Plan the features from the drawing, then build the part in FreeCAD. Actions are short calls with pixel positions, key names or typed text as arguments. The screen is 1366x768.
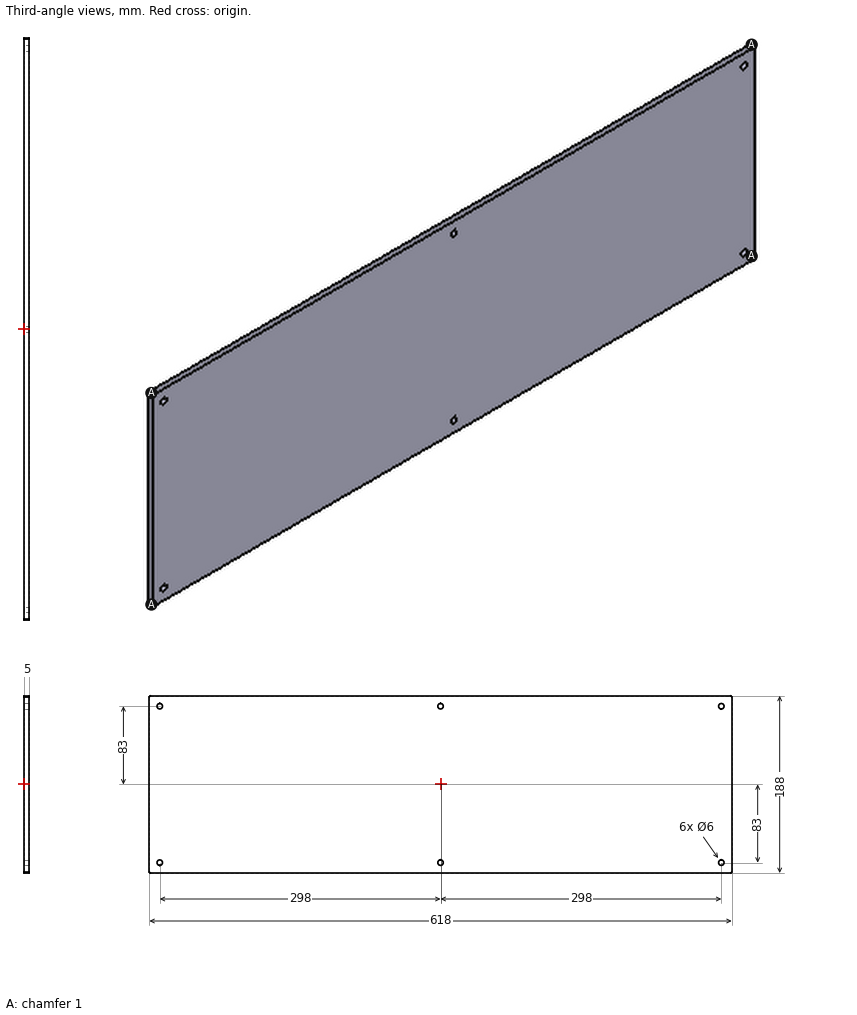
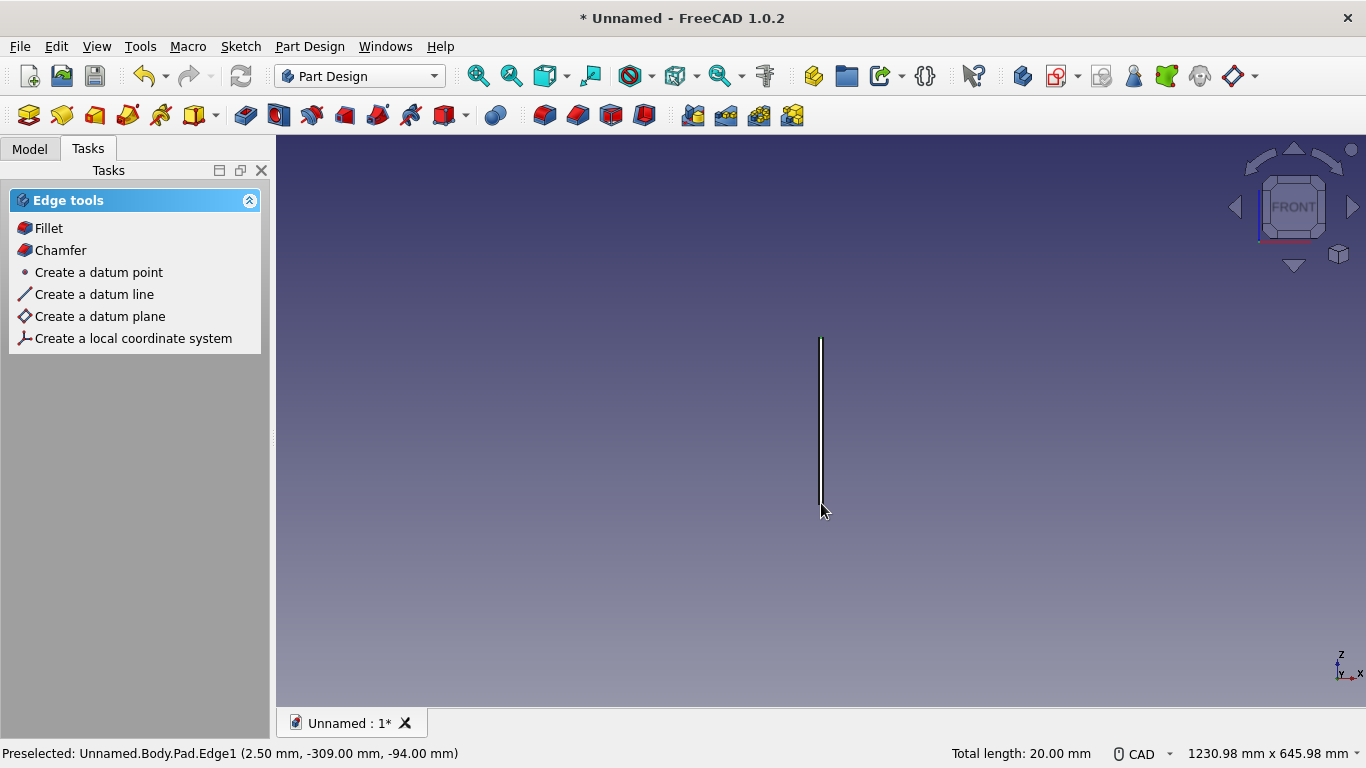
click(578, 116)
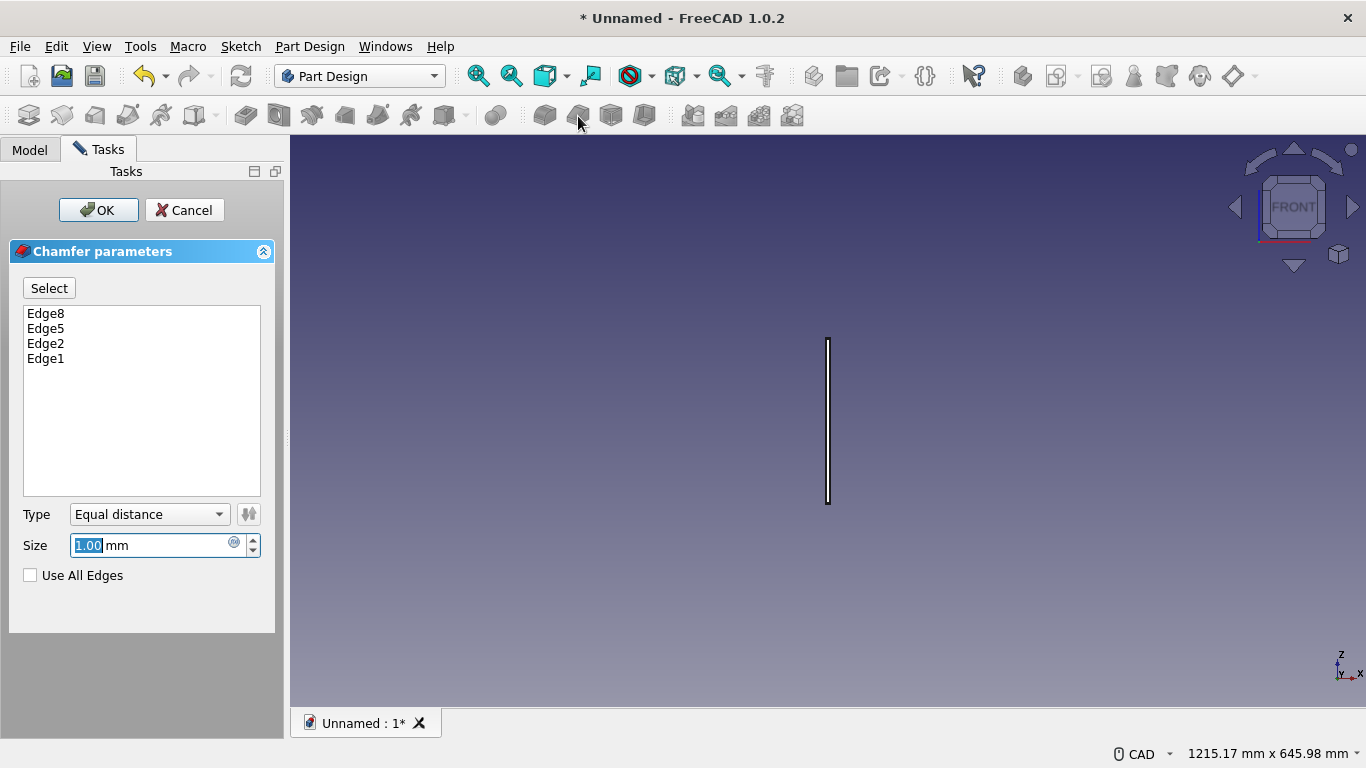
text(1)
key(Tab)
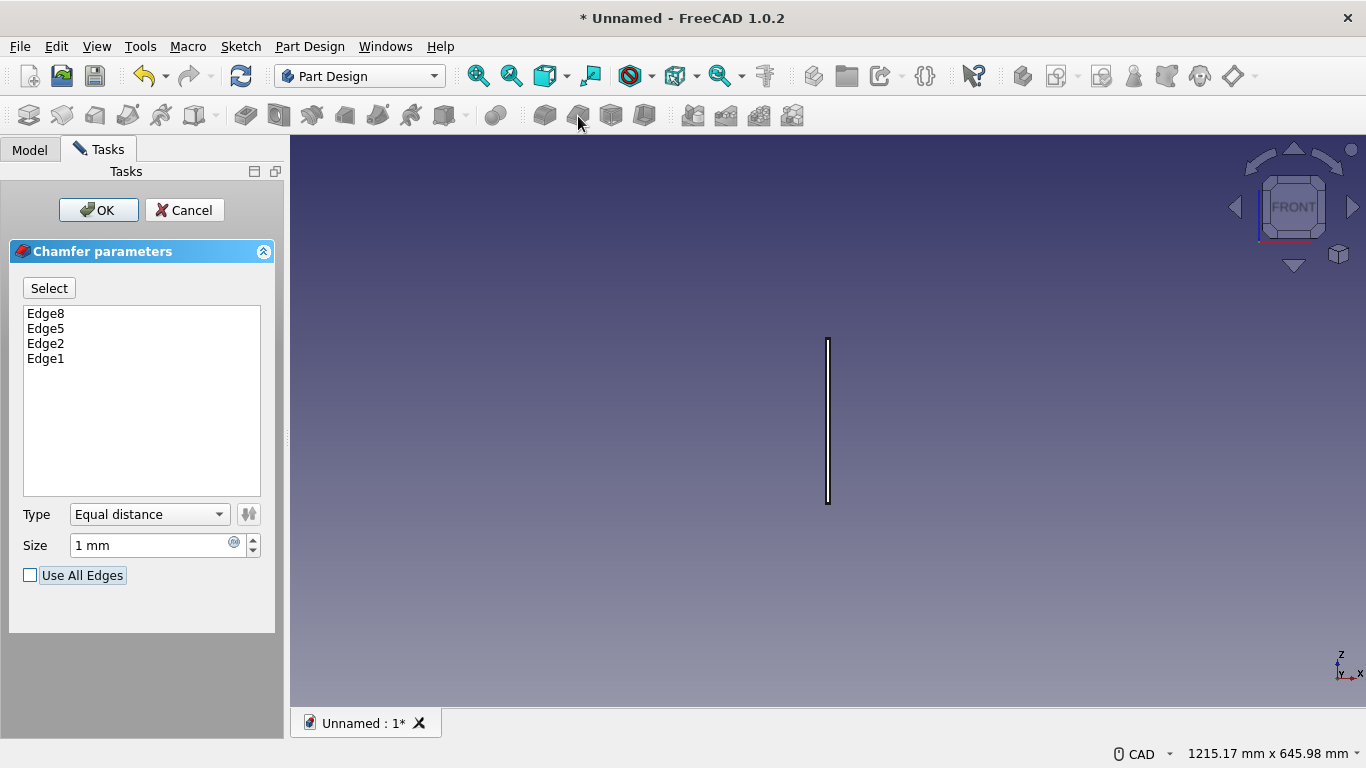
click(99, 210)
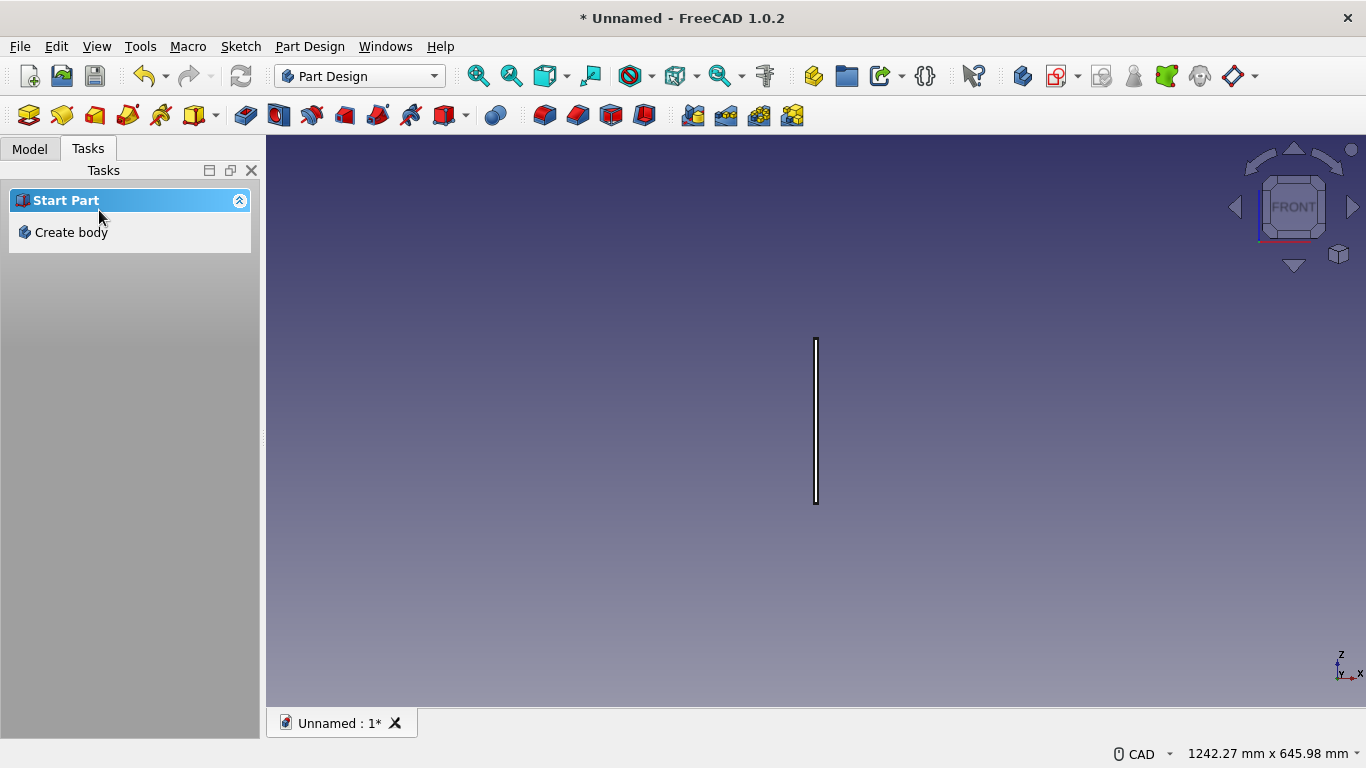
click(479, 76)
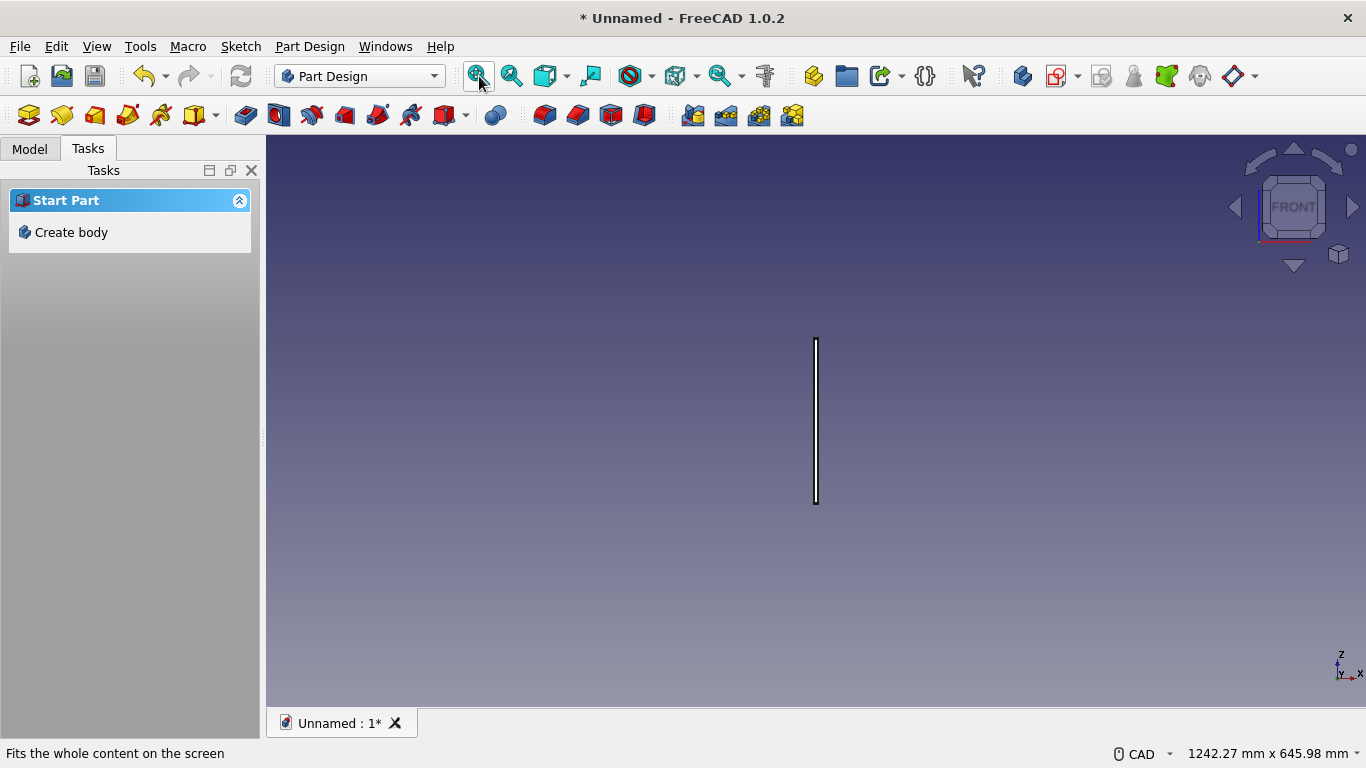
key(6)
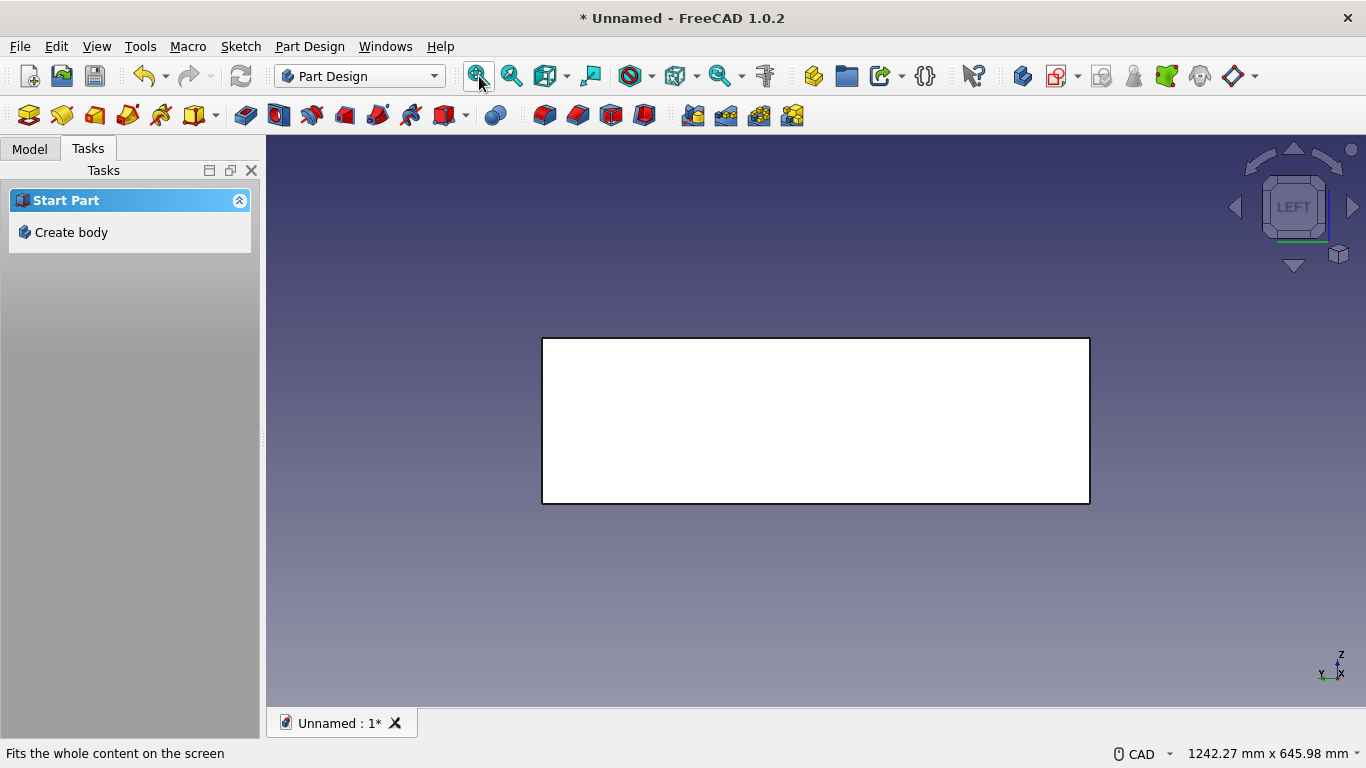
click(660, 420)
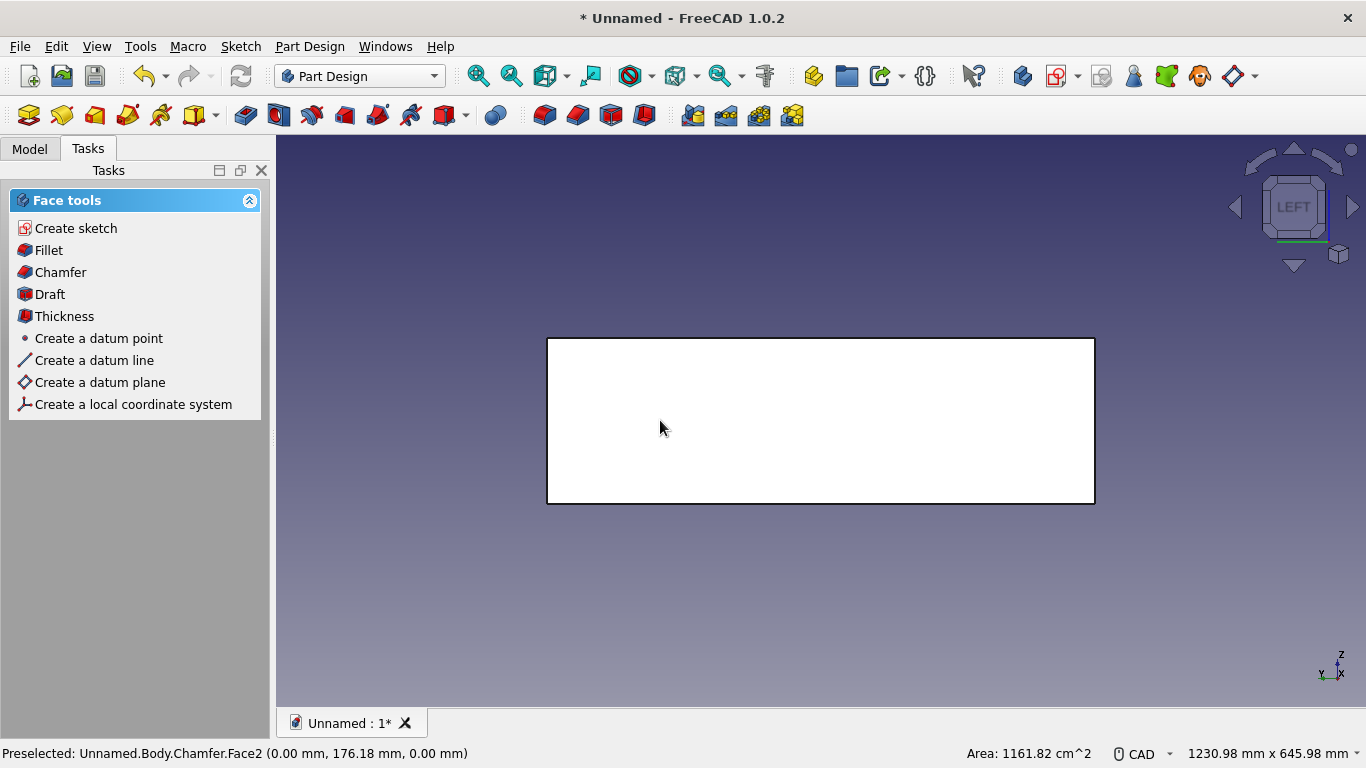
click(1056, 76)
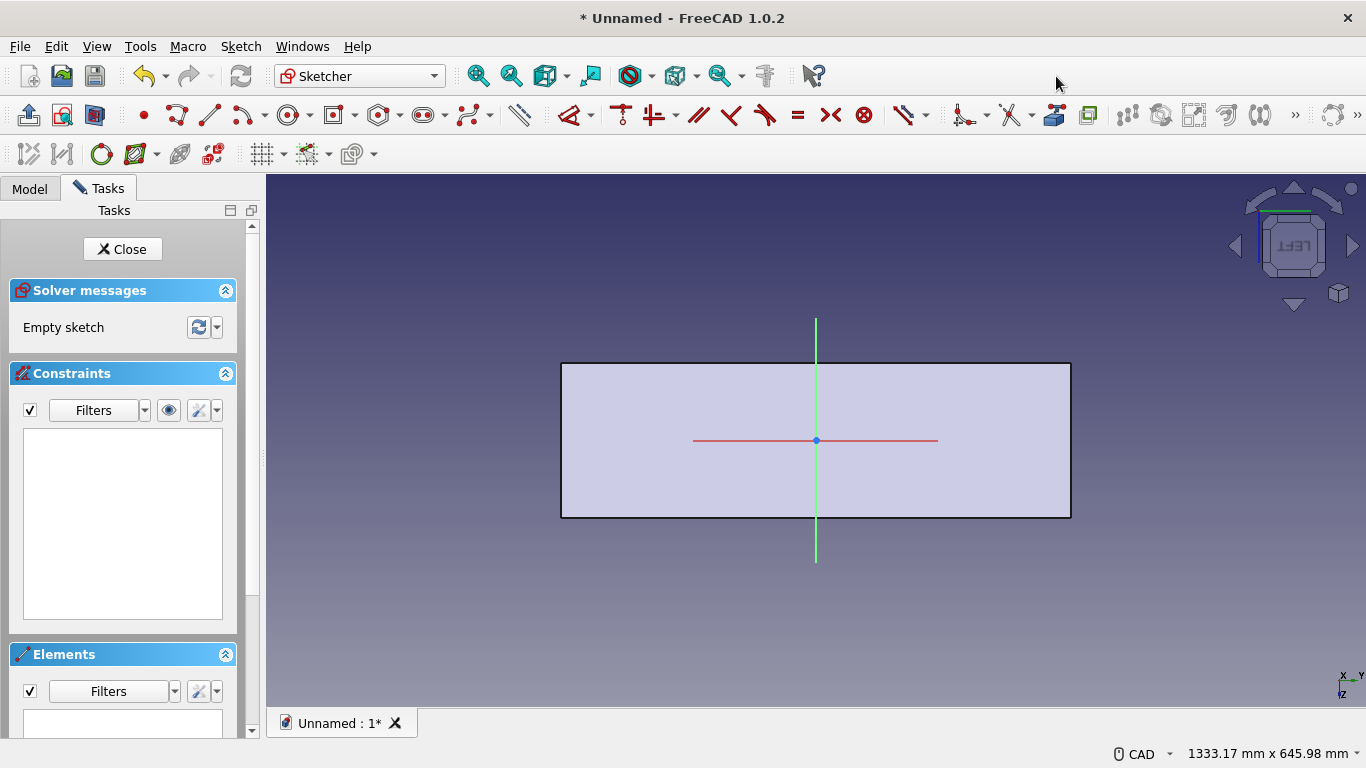
click(288, 116)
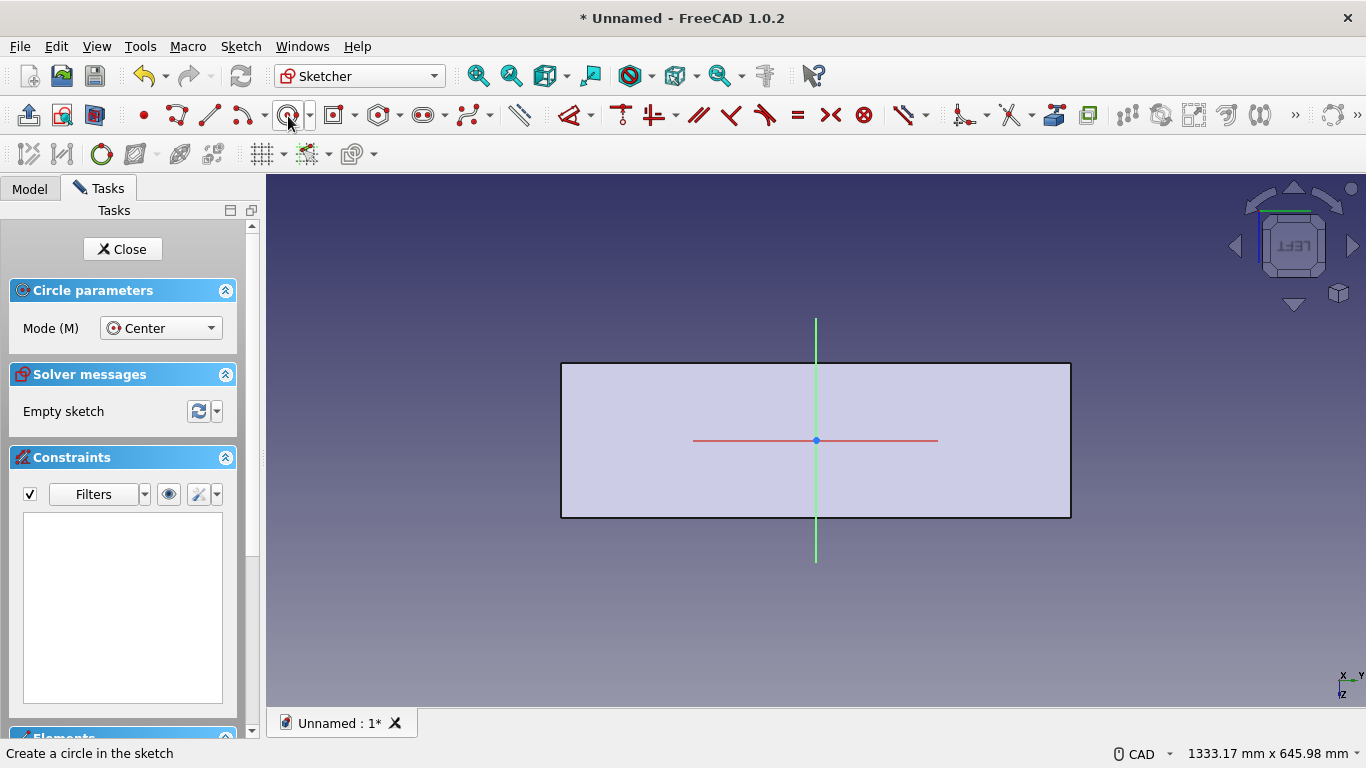
scroll(1062, 372, up, 12)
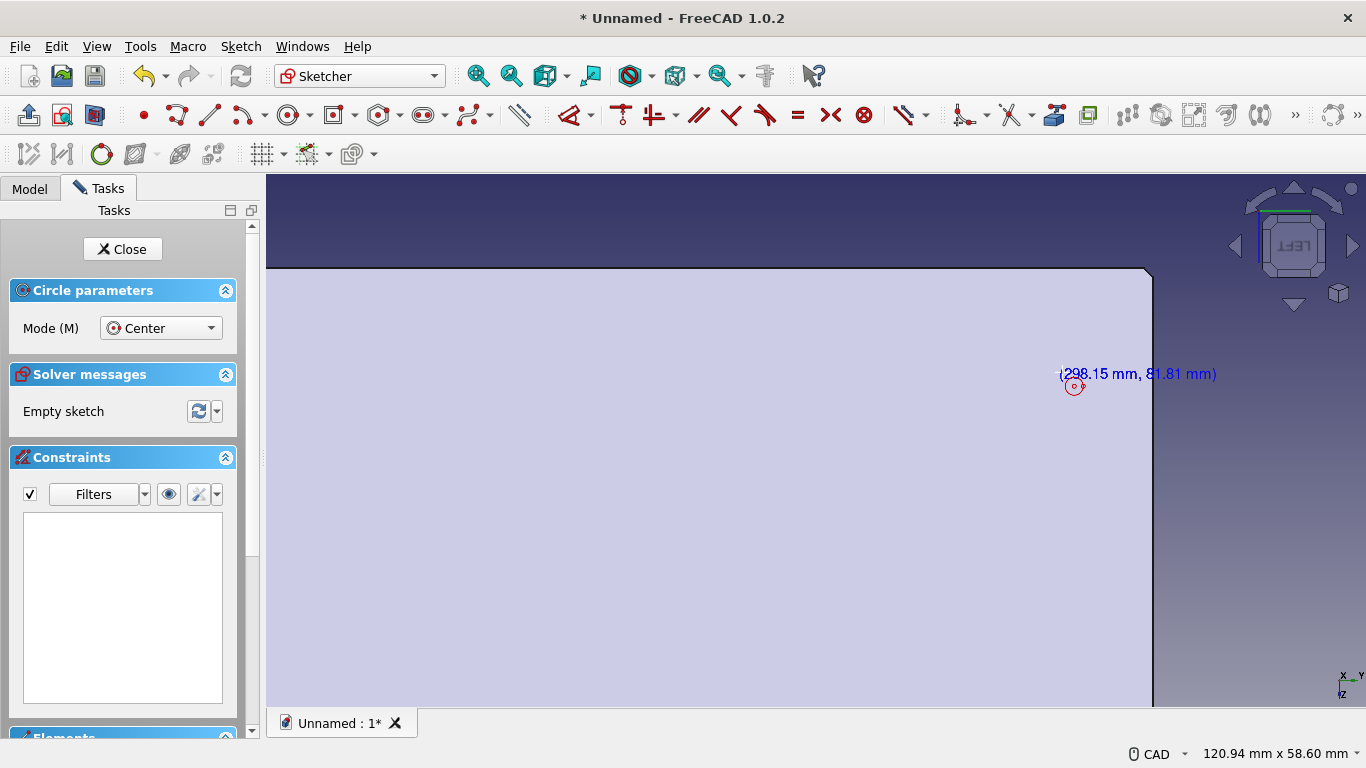
scroll(1047, 355, down, 11)